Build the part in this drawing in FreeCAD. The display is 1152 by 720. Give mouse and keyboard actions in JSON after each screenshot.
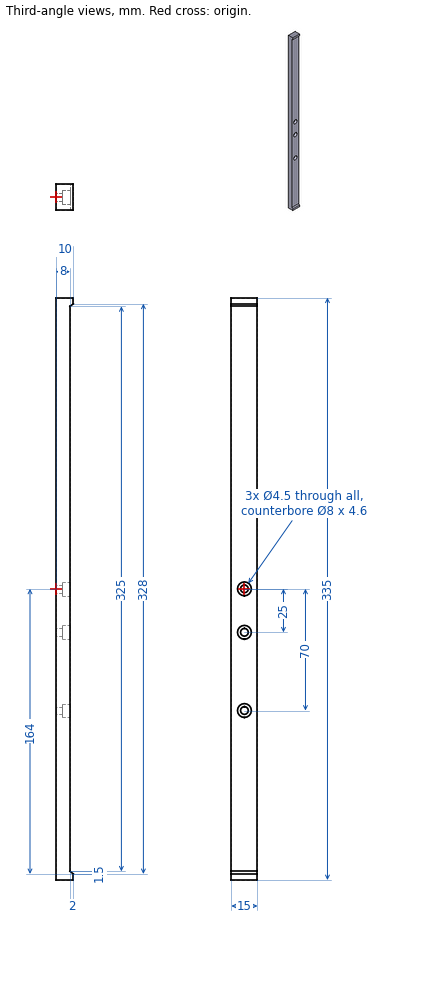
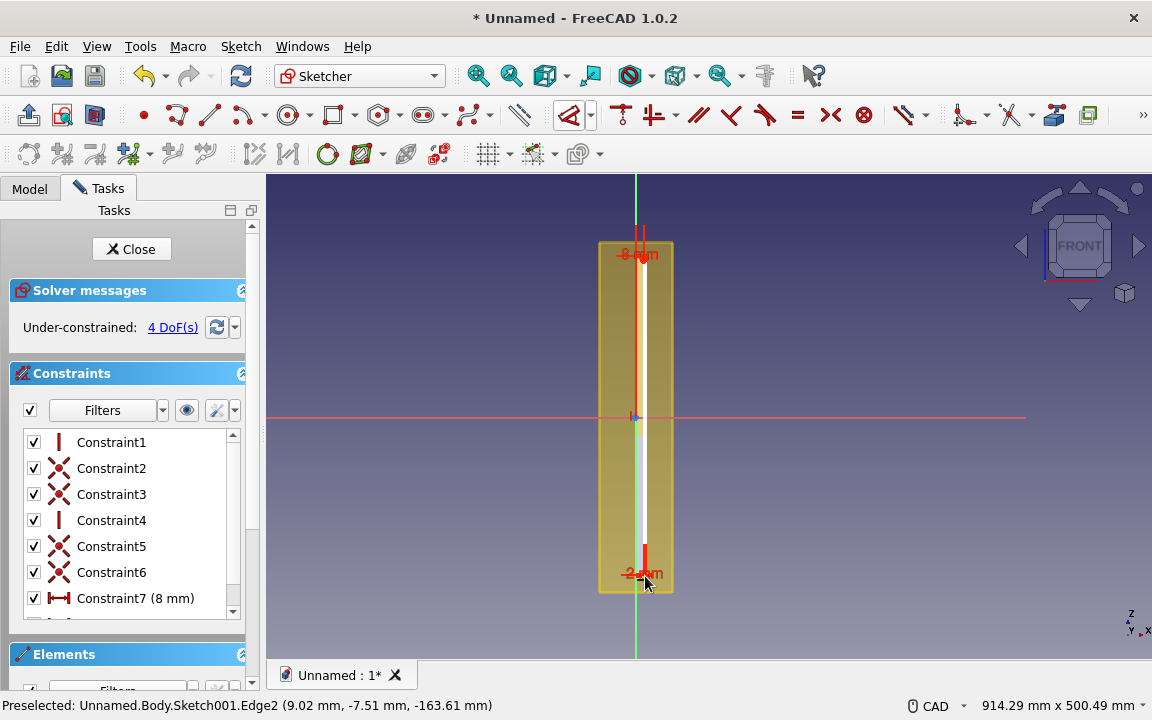
{"action": "scroll", "coordinate": [644, 355], "scroll_direction": "up", "scroll_amount": 10}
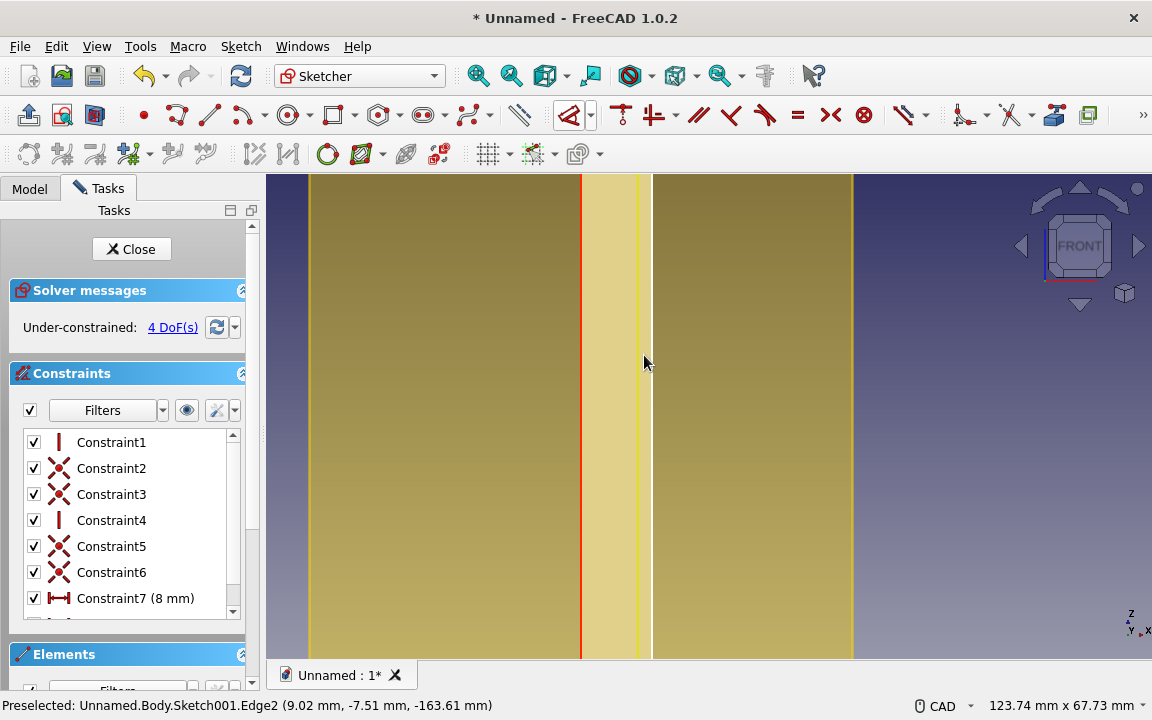
{"action": "left_click", "coordinate": [638, 354]}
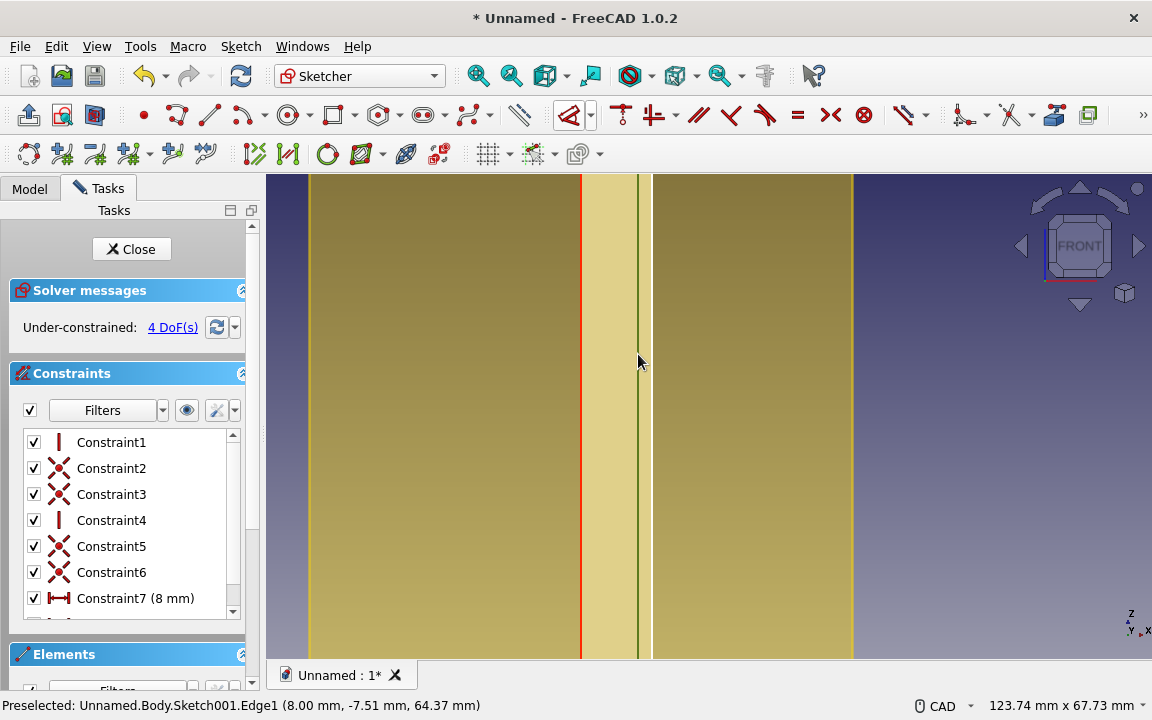
{"action": "left_click", "coordinate": [590, 116]}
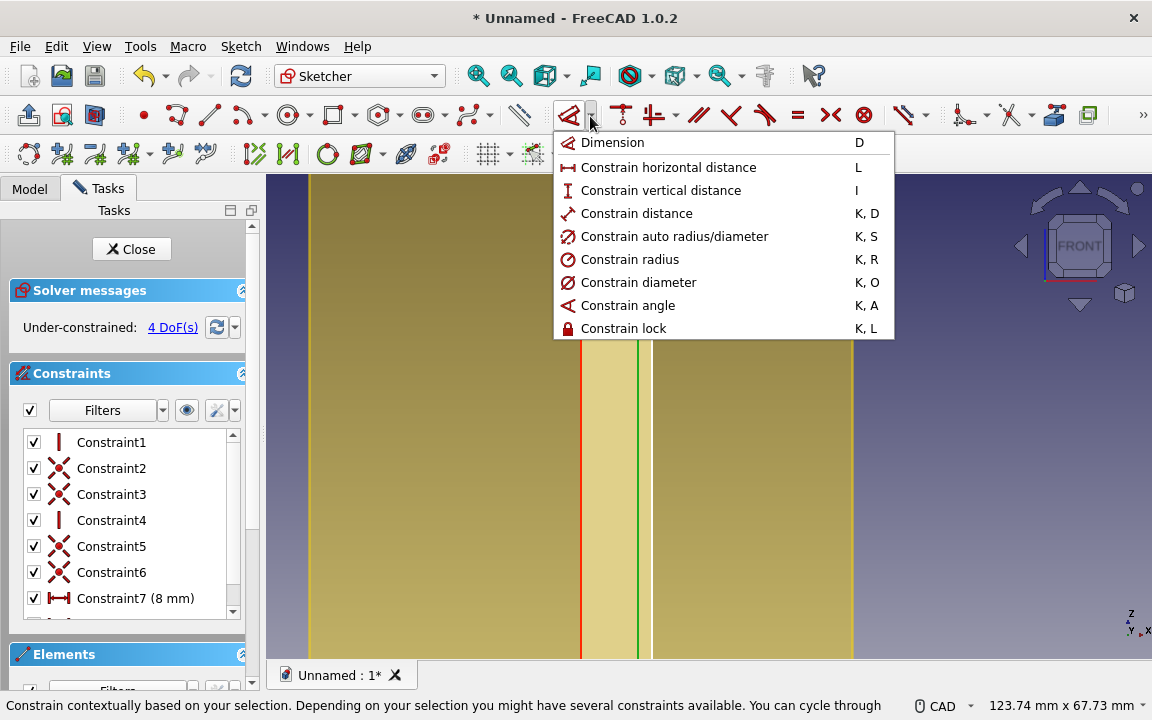
{"action": "left_click", "coordinate": [724, 190]}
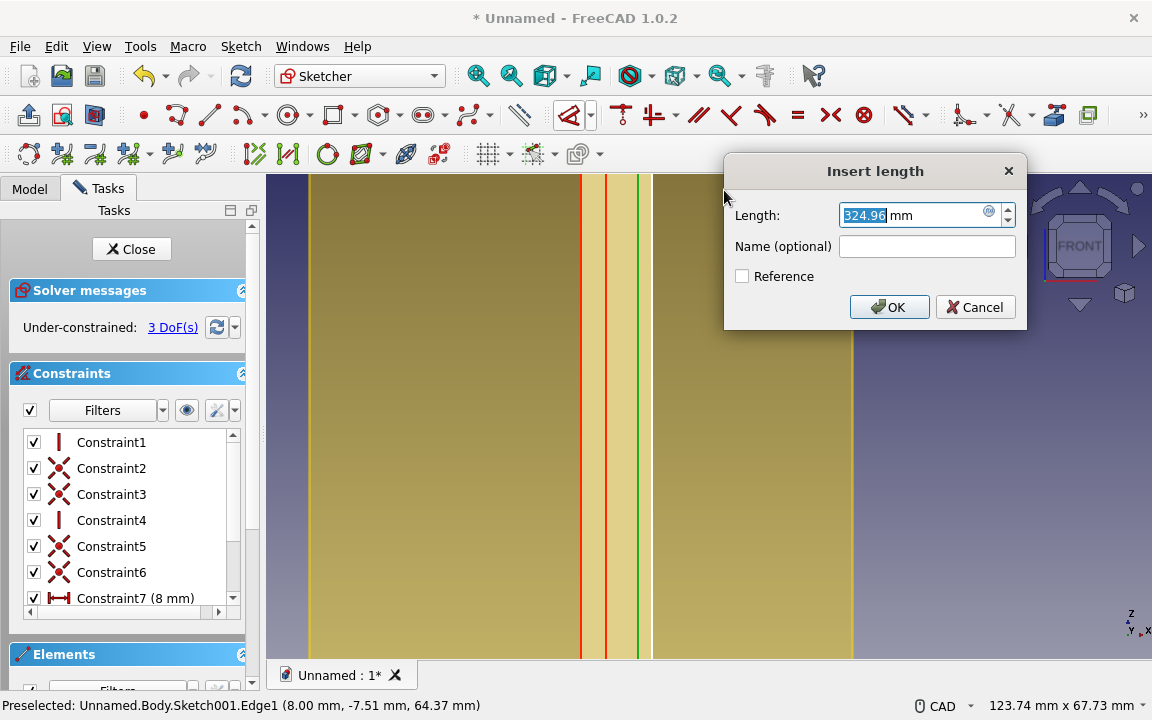
{"action": "type", "text": "325"}
{"action": "key", "text": "Return"}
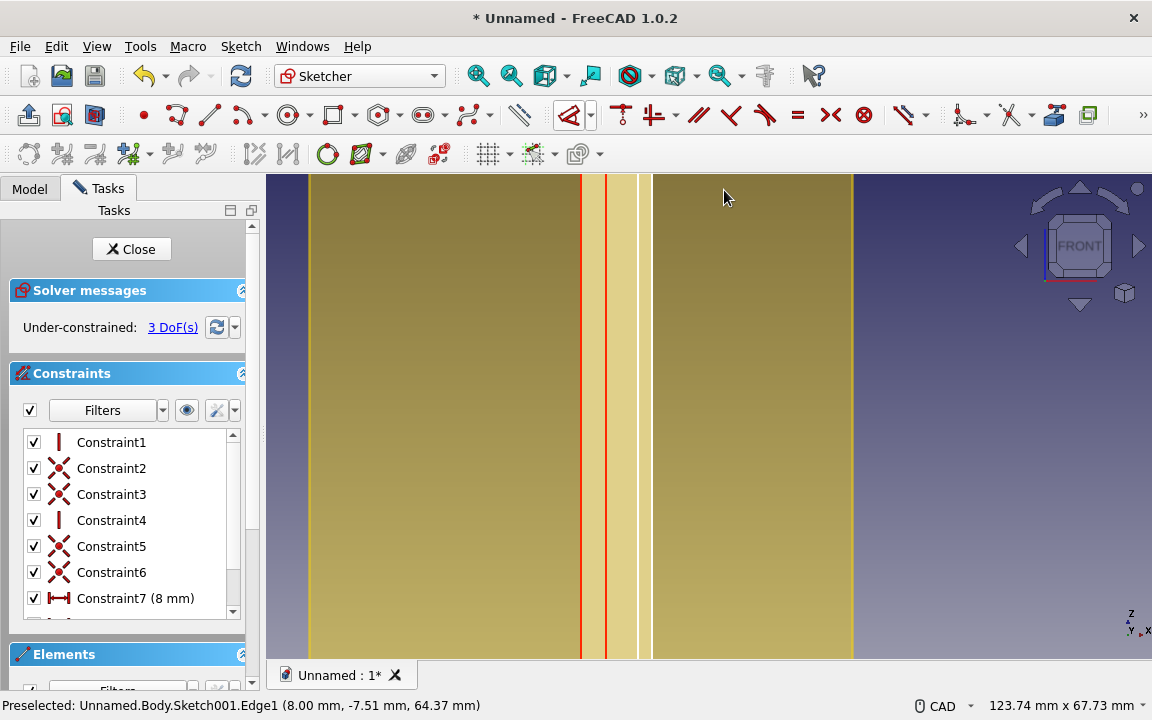
{"action": "left_click", "coordinate": [652, 347]}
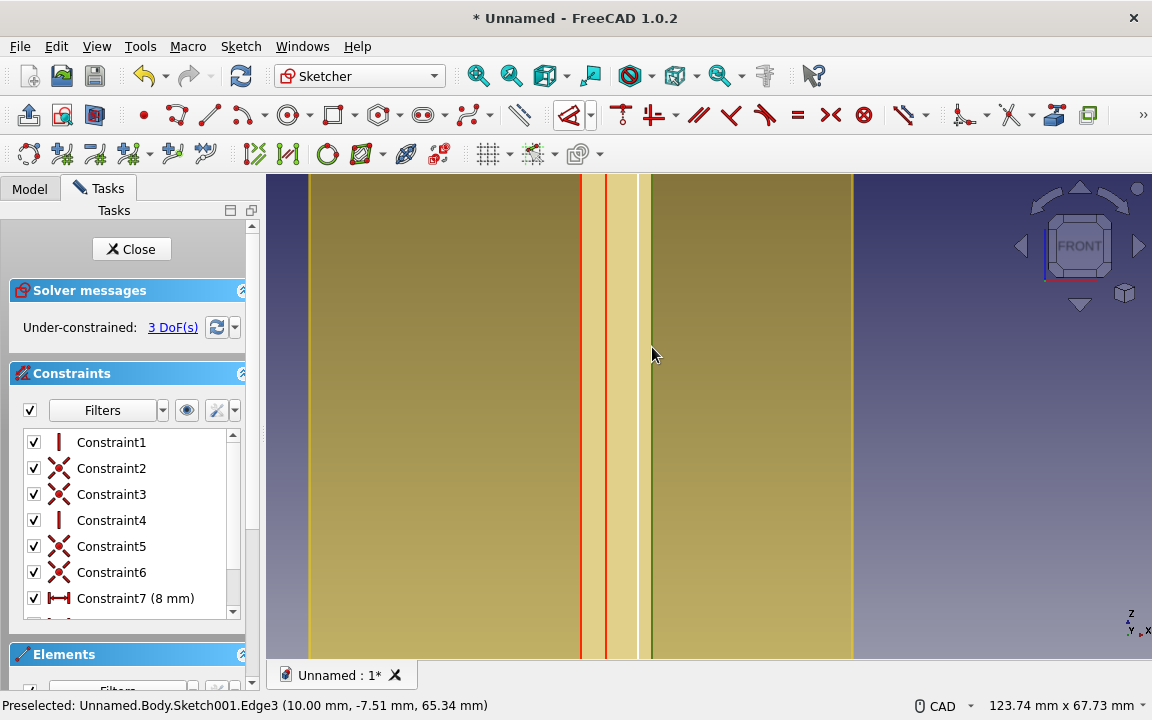
{"action": "left_click", "coordinate": [590, 116]}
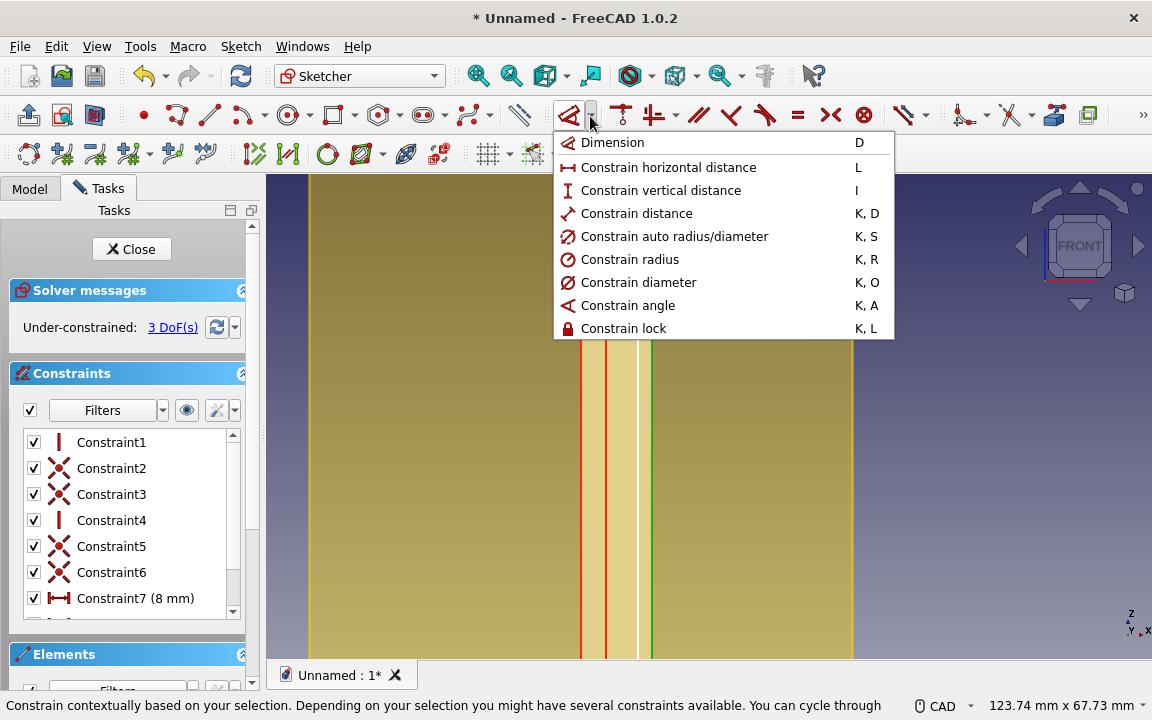
{"action": "left_click", "coordinate": [724, 190]}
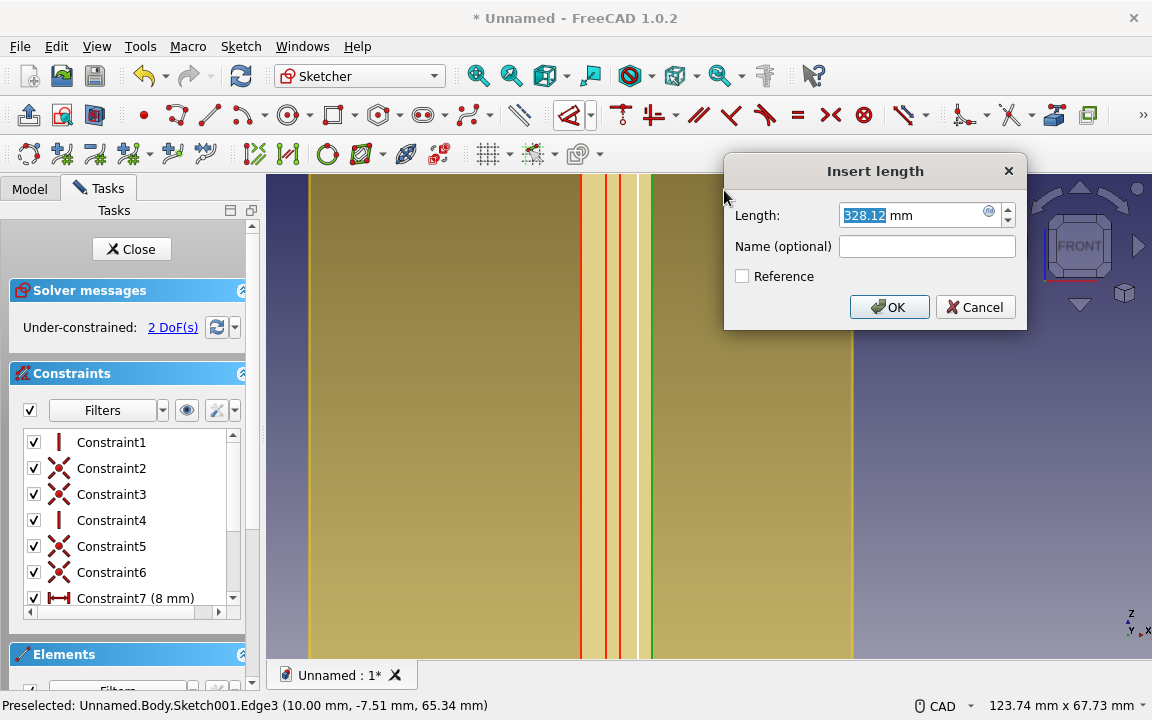
{"action": "type", "text": "328"}
{"action": "key", "text": "Return"}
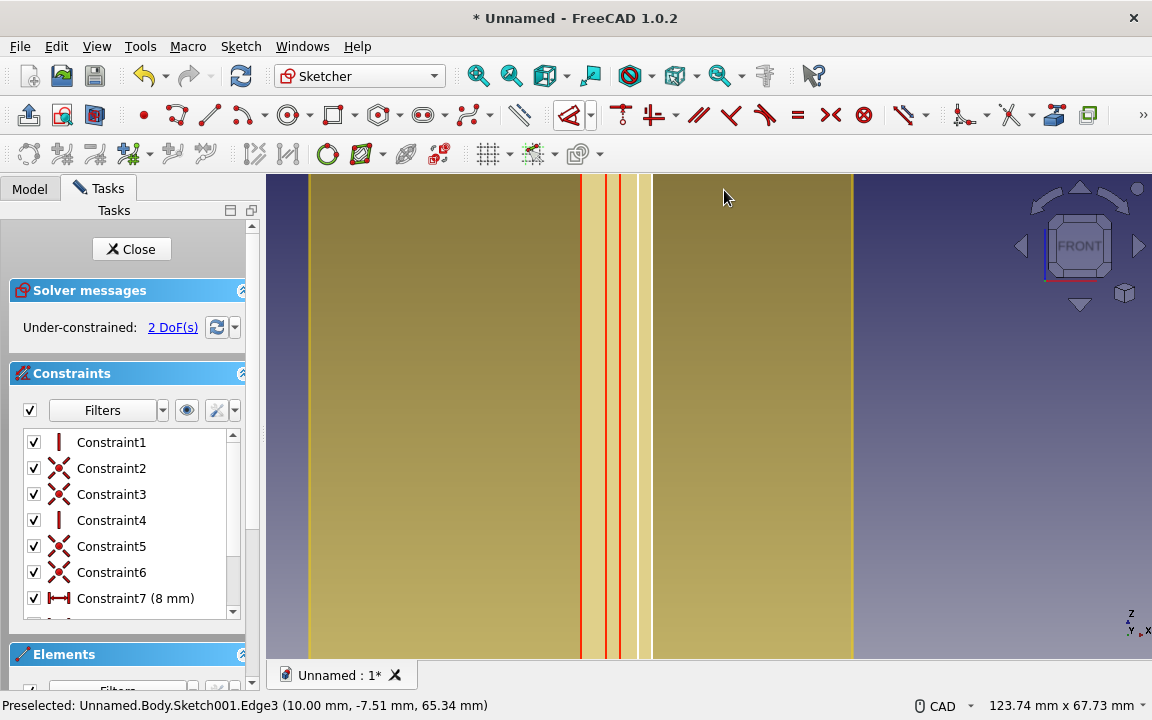
{"action": "scroll", "coordinate": [644, 354], "scroll_direction": "down", "scroll_amount": 10}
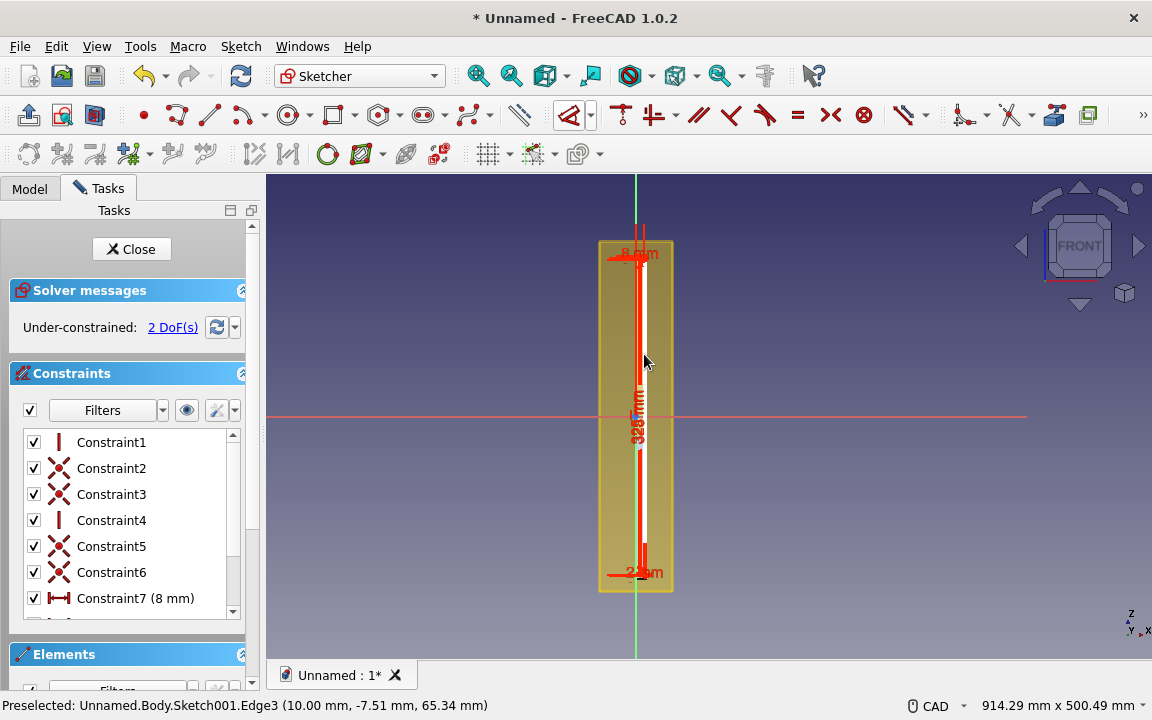
{"action": "scroll", "coordinate": [646, 576], "scroll_direction": "up", "scroll_amount": 9}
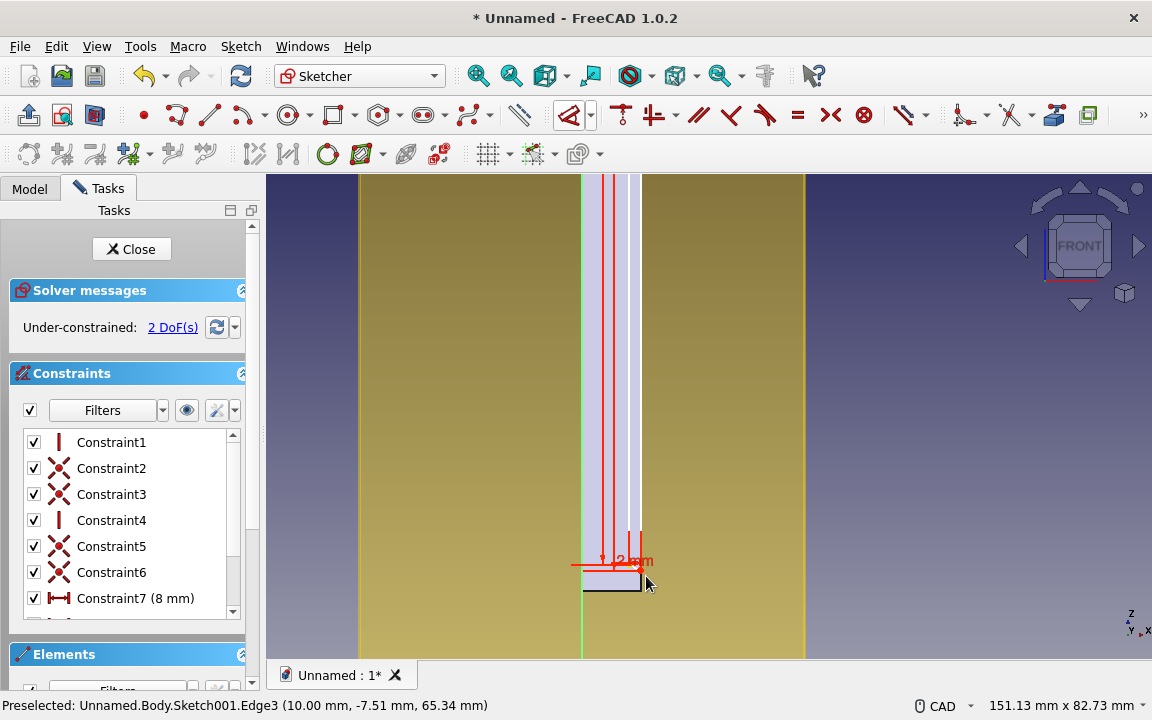
{"action": "left_click", "coordinate": [641, 571]}